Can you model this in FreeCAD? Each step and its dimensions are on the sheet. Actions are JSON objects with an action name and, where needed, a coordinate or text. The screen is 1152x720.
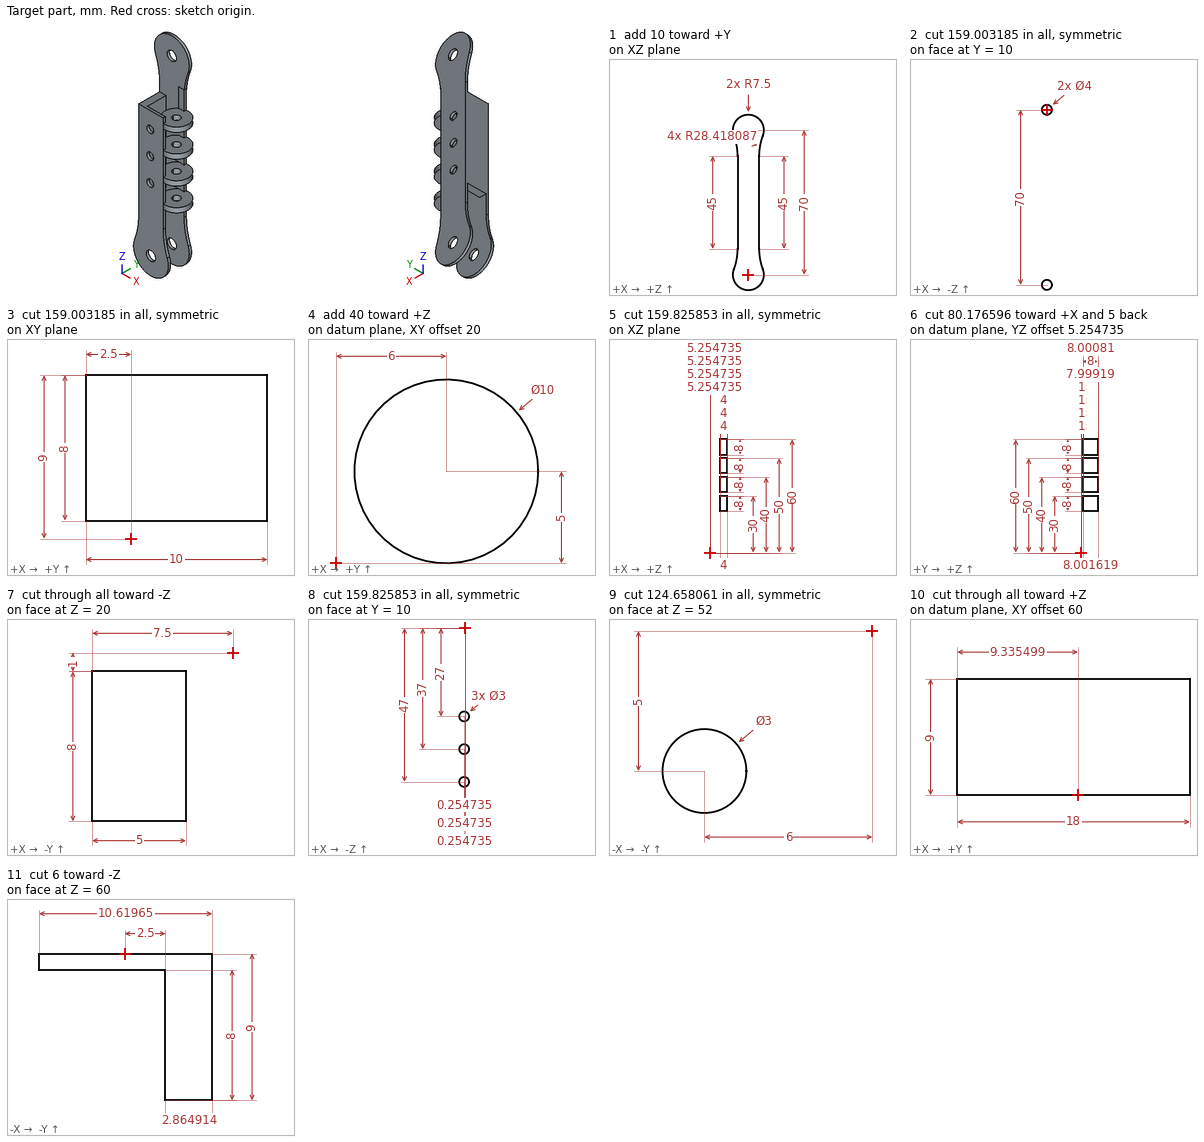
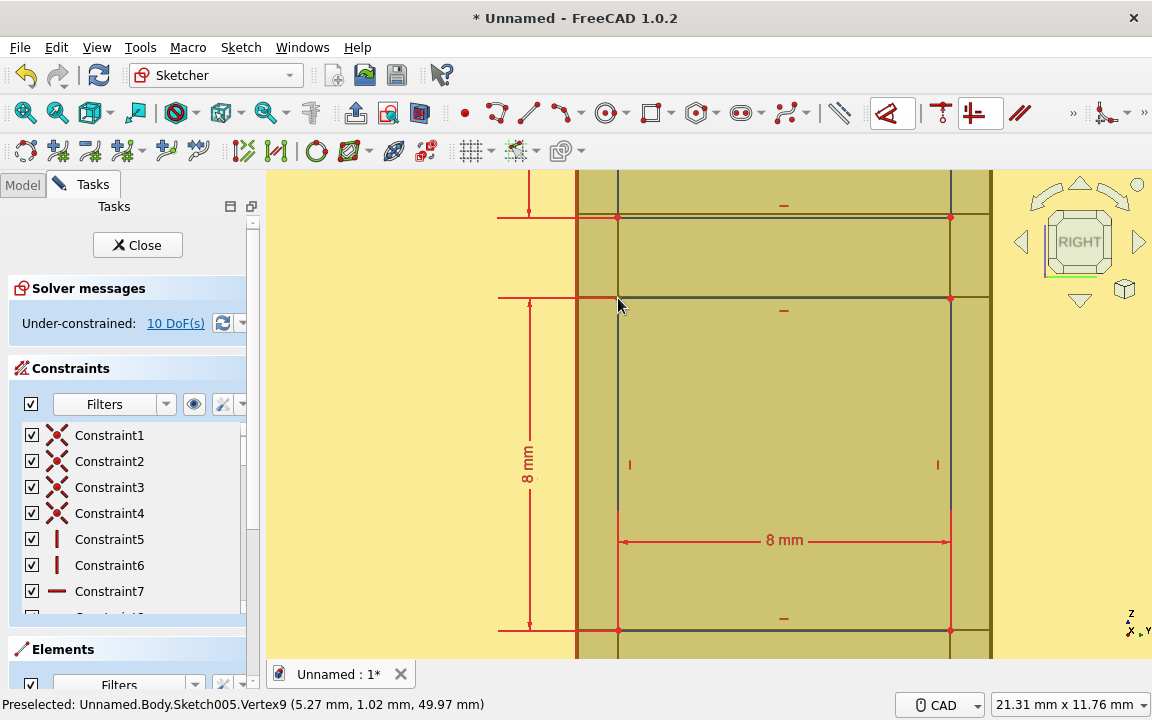
{"action": "key", "text": "l"}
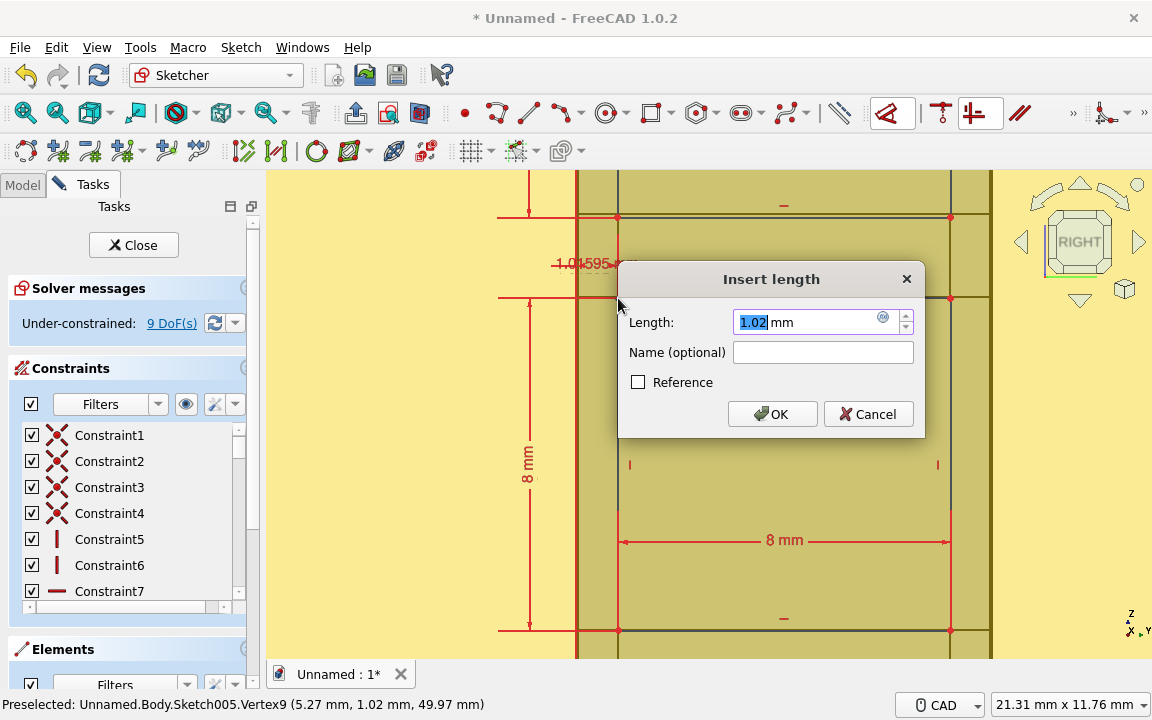
{"action": "type", "text": "1"}
{"action": "key", "text": "Return"}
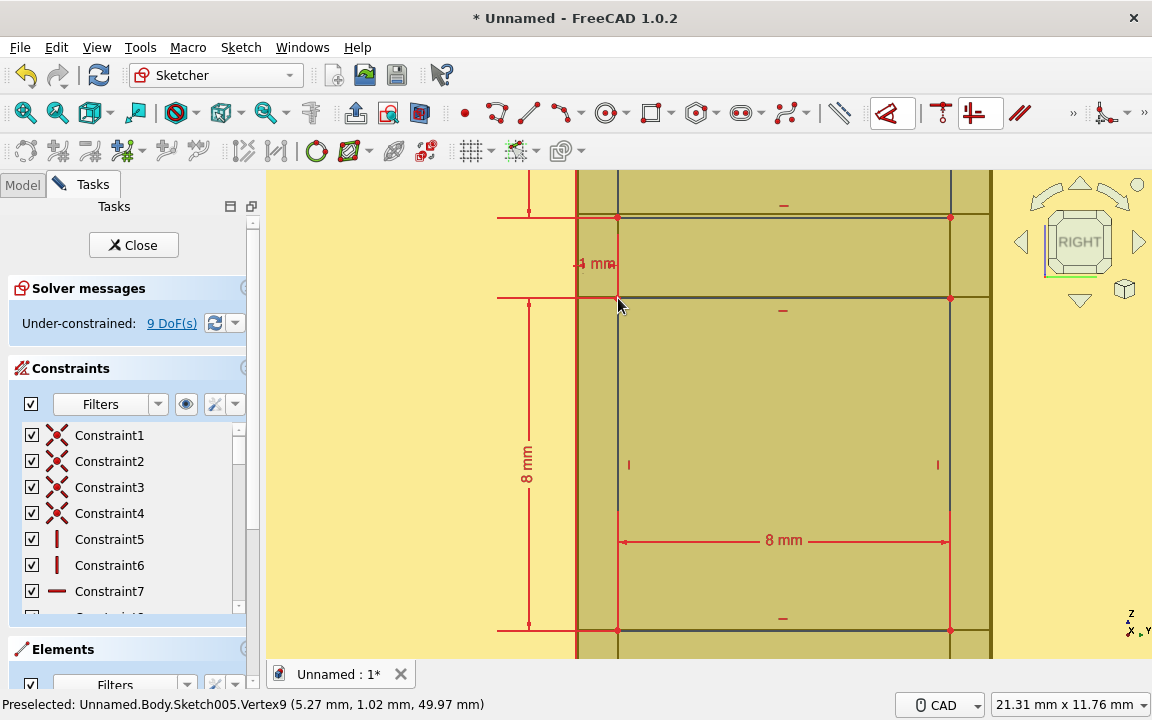
{"action": "scroll", "coordinate": [621, 303], "scroll_direction": "down", "scroll_amount": 10}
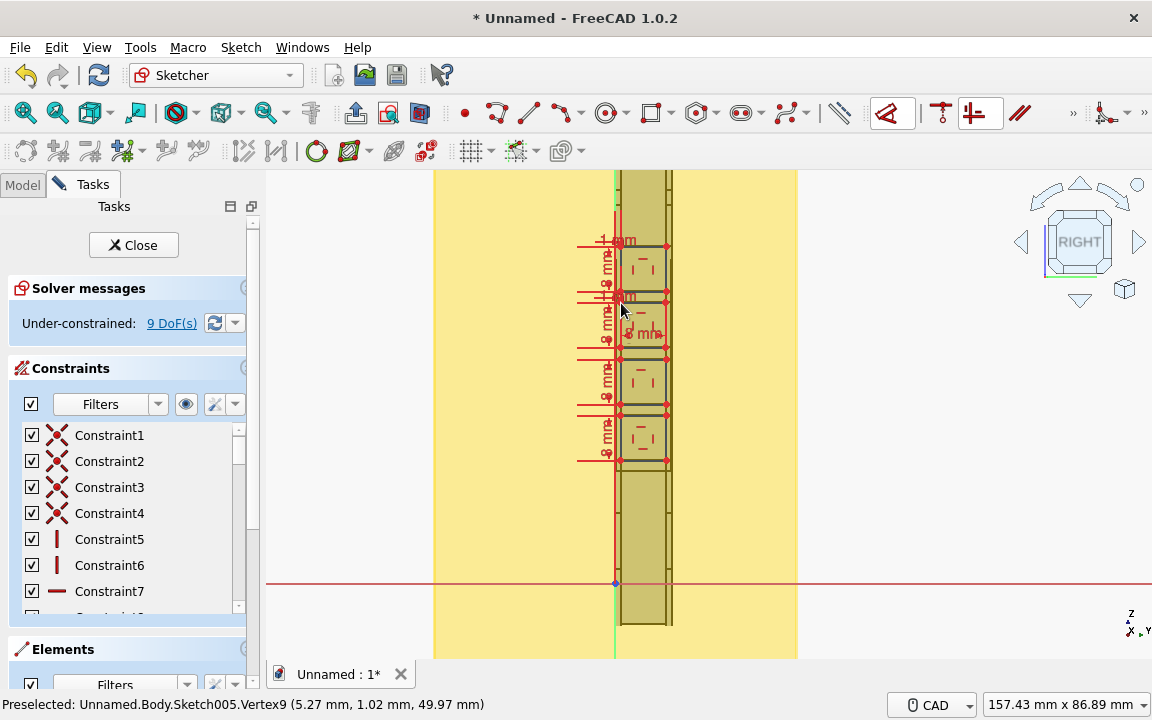
{"action": "scroll", "coordinate": [621, 360], "scroll_direction": "up", "scroll_amount": 10}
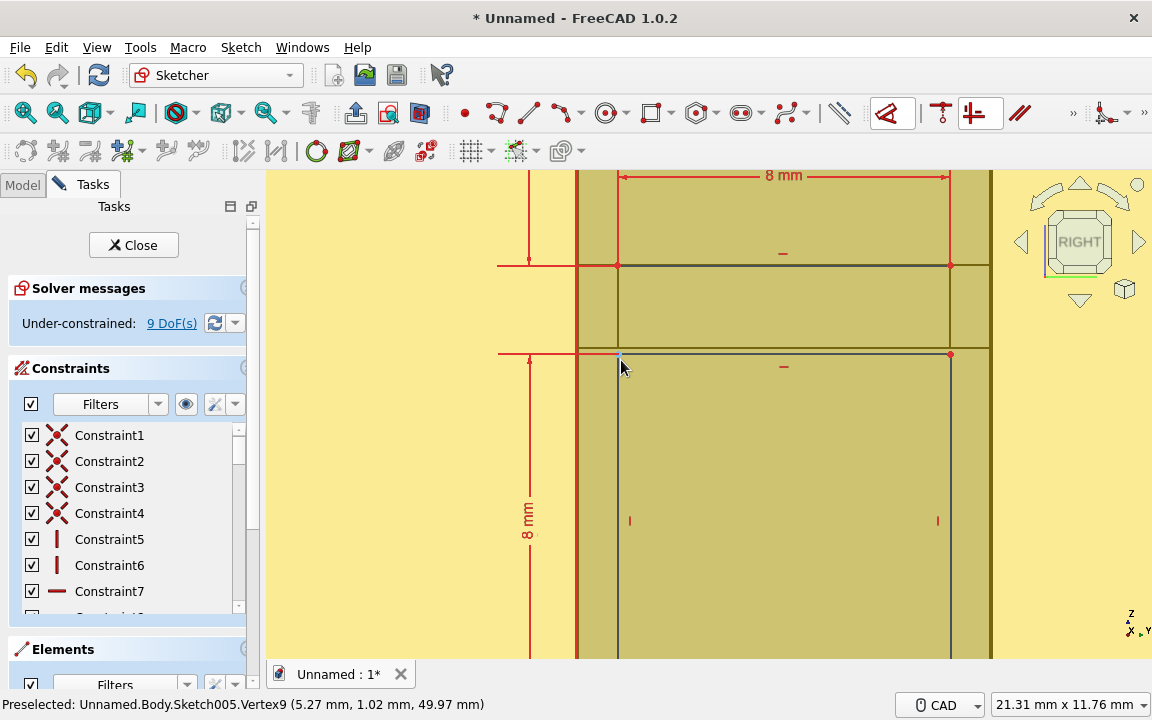
{"action": "left_click", "coordinate": [618, 354]}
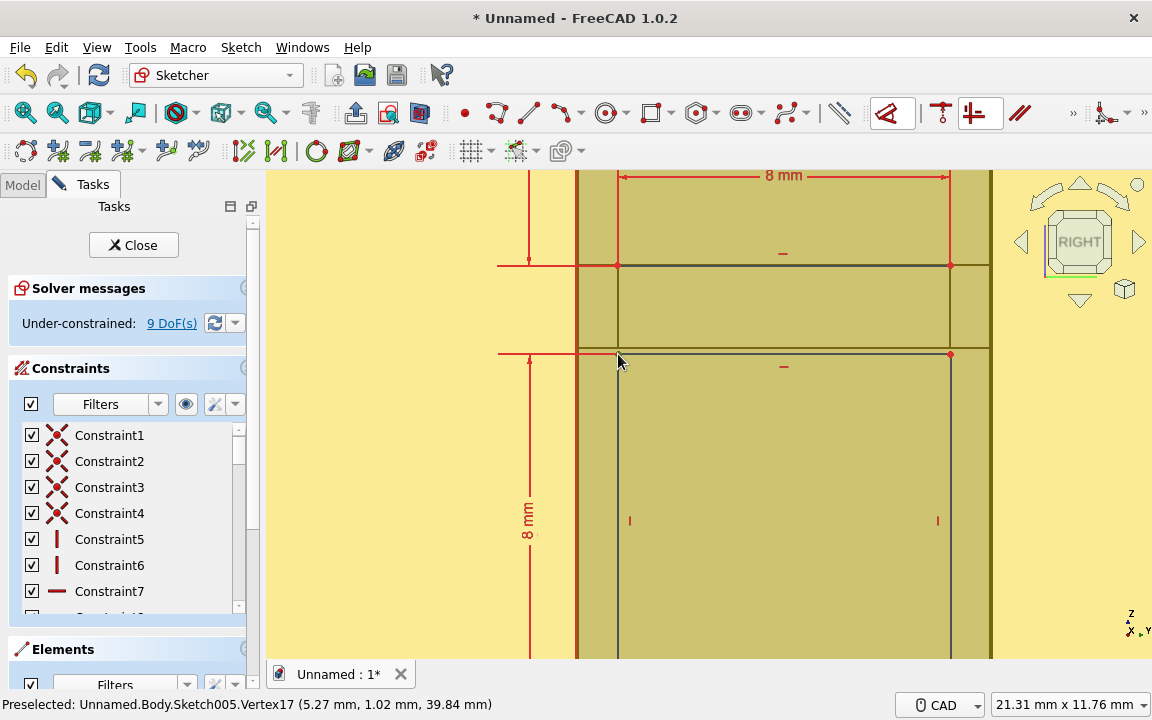
{"action": "left_click", "coordinate": [910, 114]}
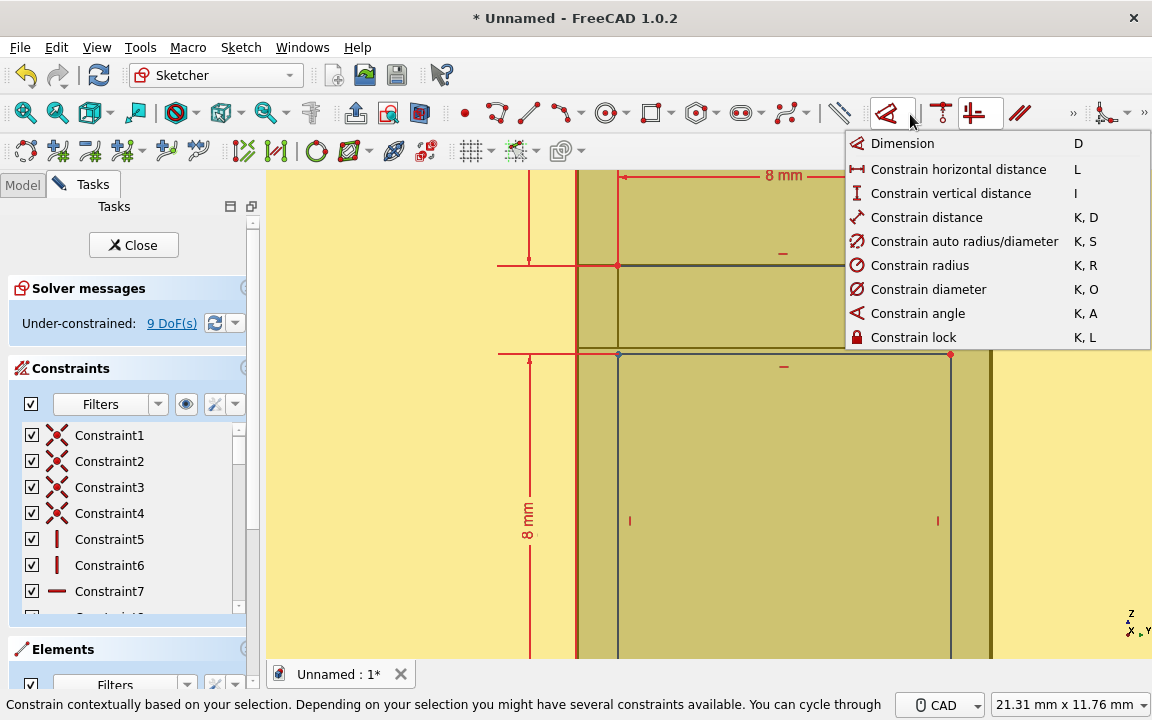
{"action": "left_click", "coordinate": [998, 169]}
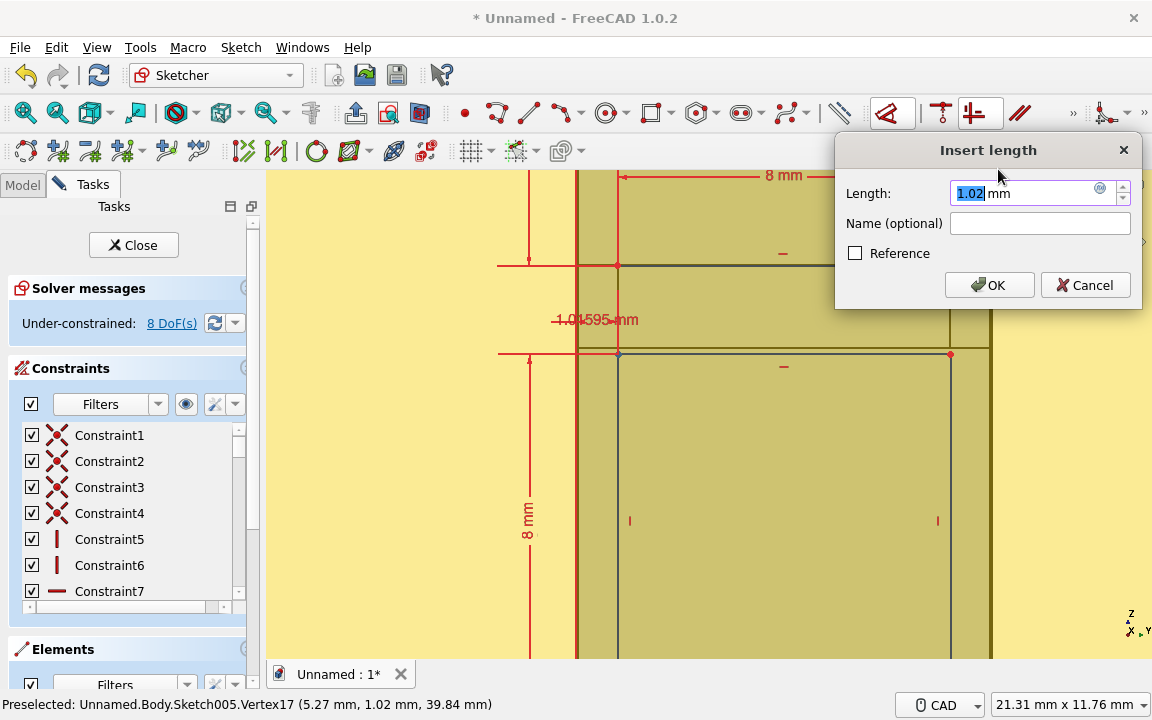
{"action": "type", "text": "1"}
{"action": "key", "text": "Return"}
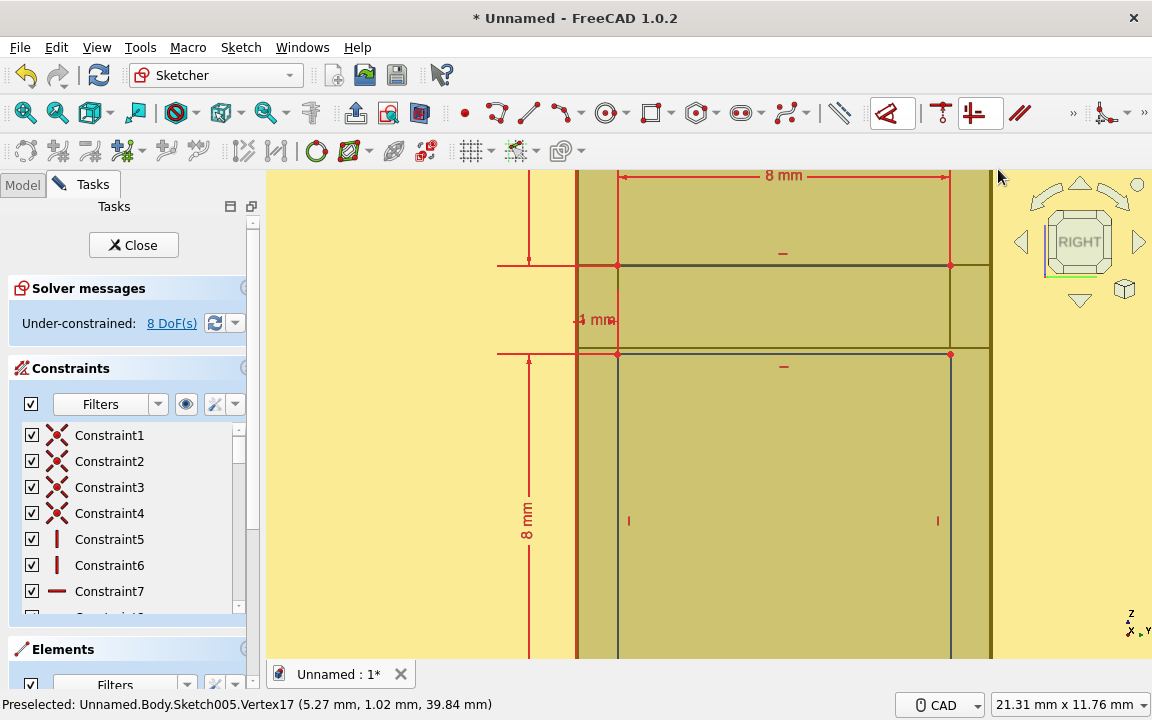
{"action": "scroll", "coordinate": [621, 360], "scroll_direction": "down", "scroll_amount": 10}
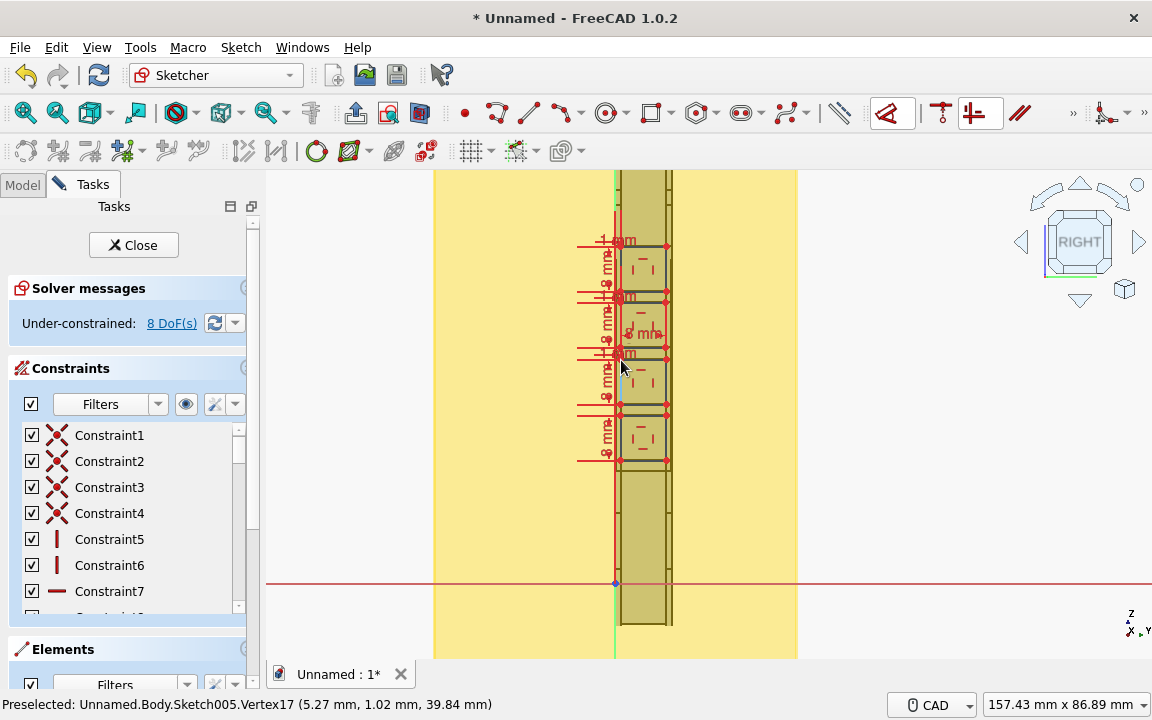
{"action": "scroll", "coordinate": [621, 416], "scroll_direction": "up", "scroll_amount": 10}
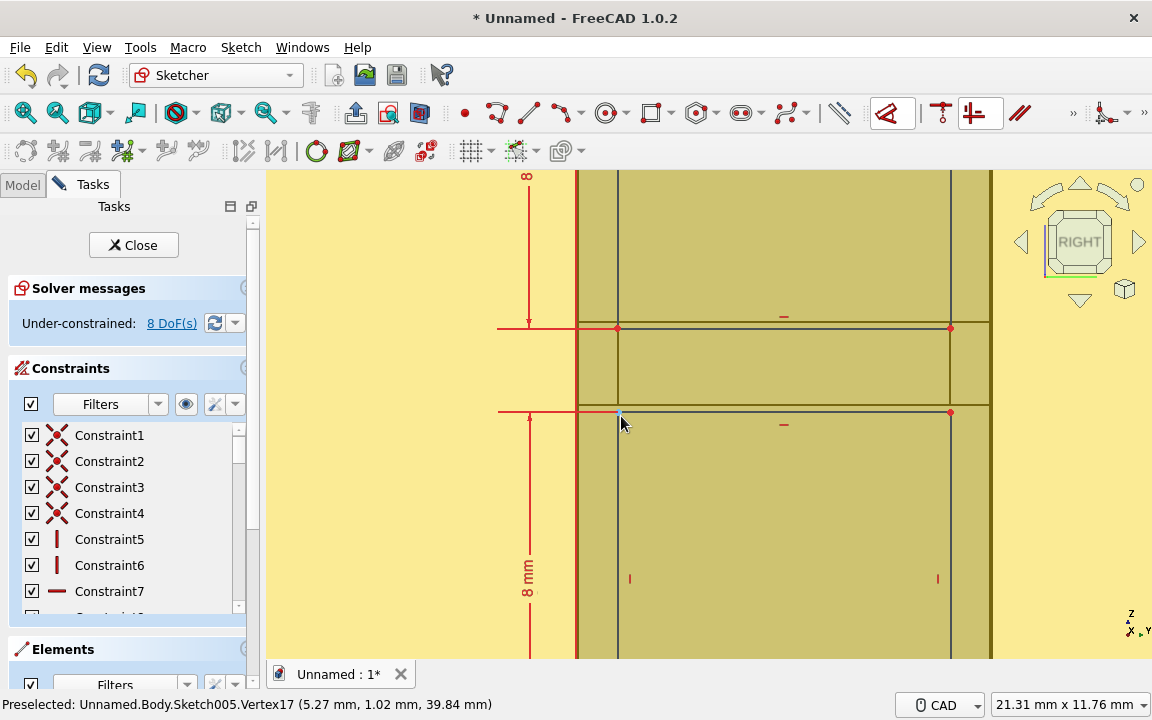
{"action": "left_click", "coordinate": [618, 412]}